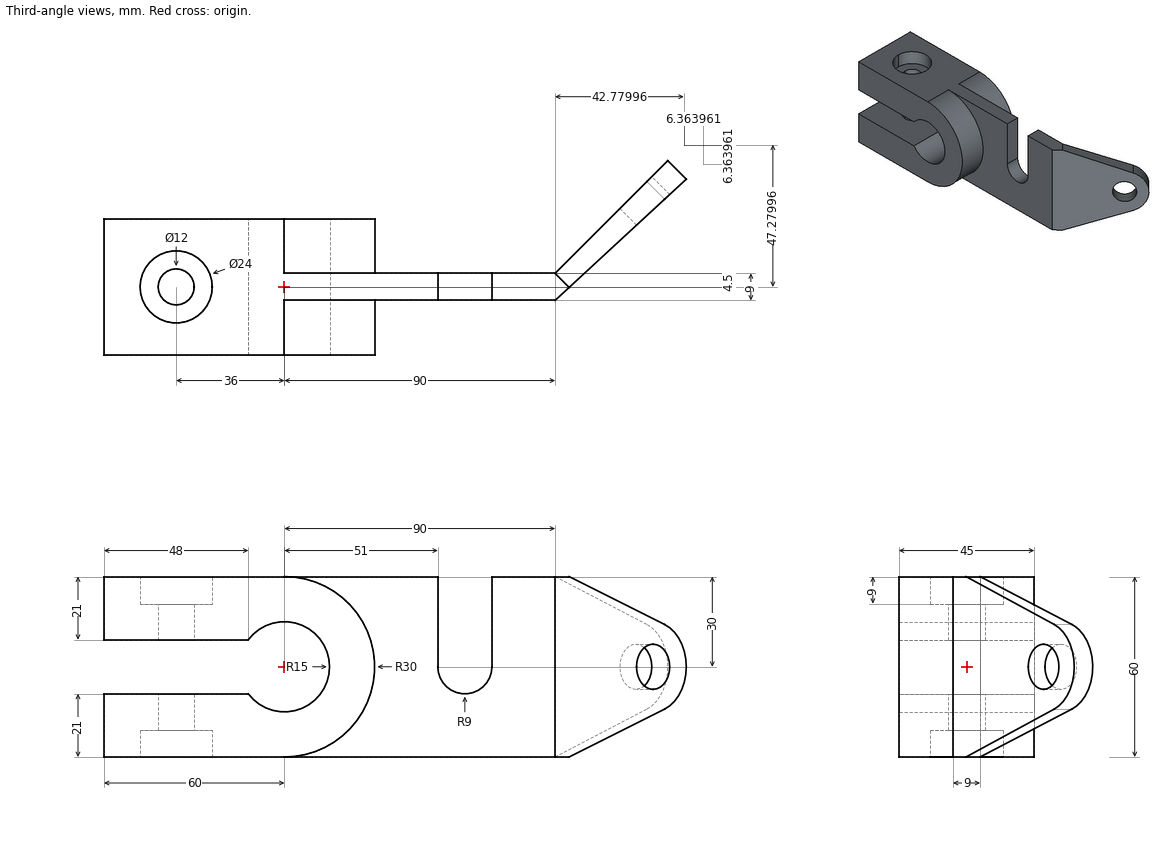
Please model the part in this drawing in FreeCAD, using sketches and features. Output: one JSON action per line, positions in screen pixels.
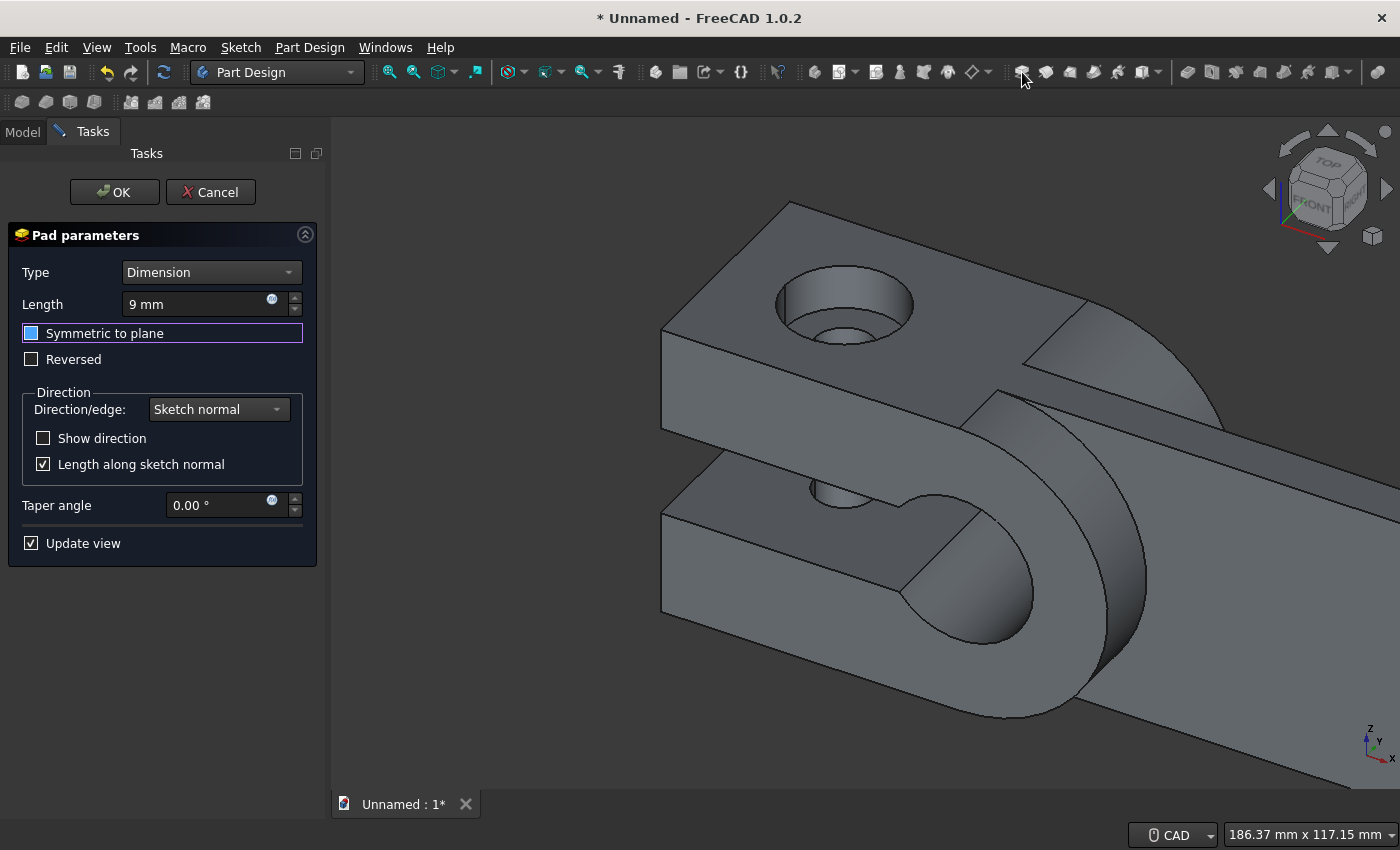
{"action": "left_click", "coordinate": [30, 333]}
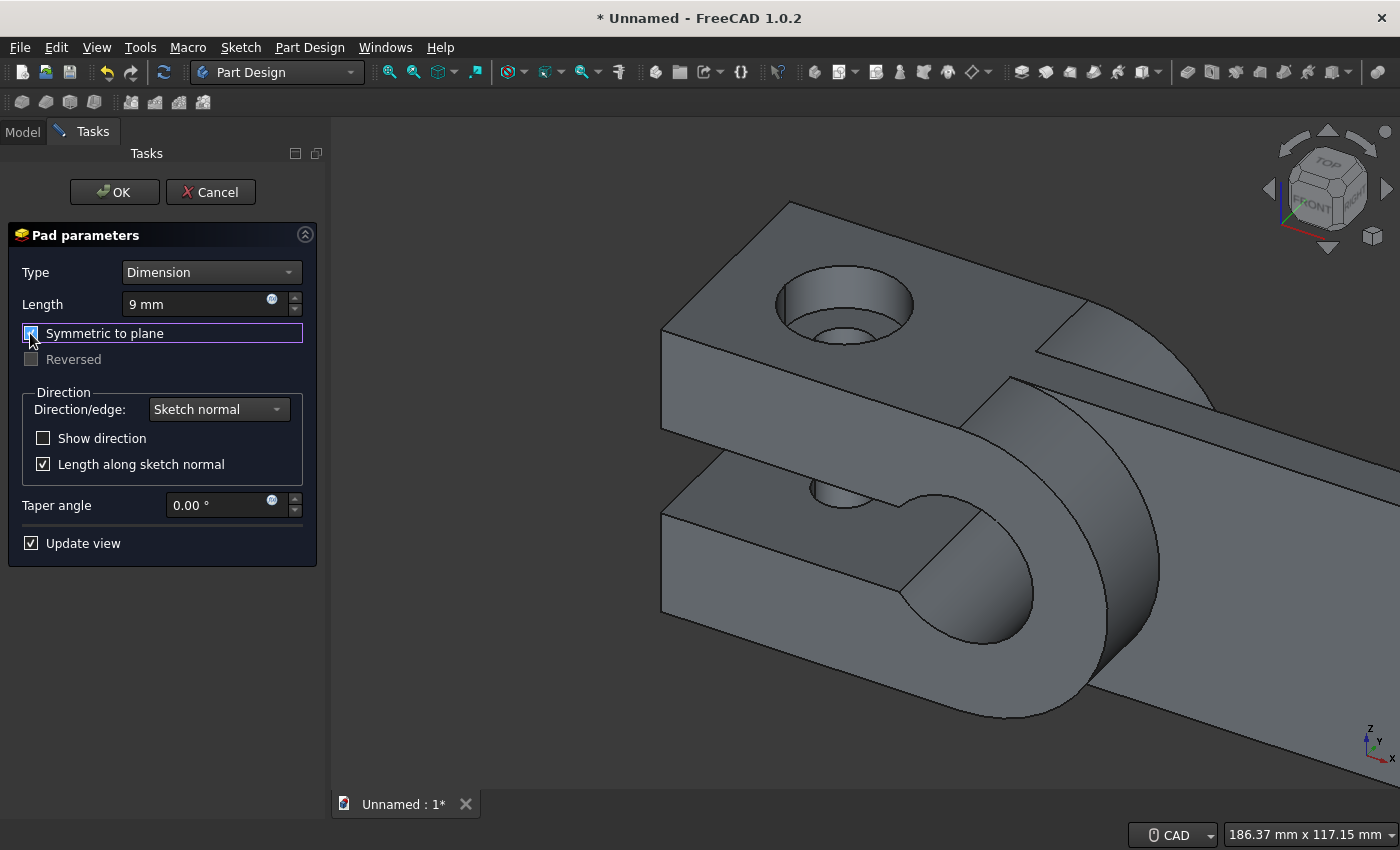
{"action": "left_click", "coordinate": [115, 192]}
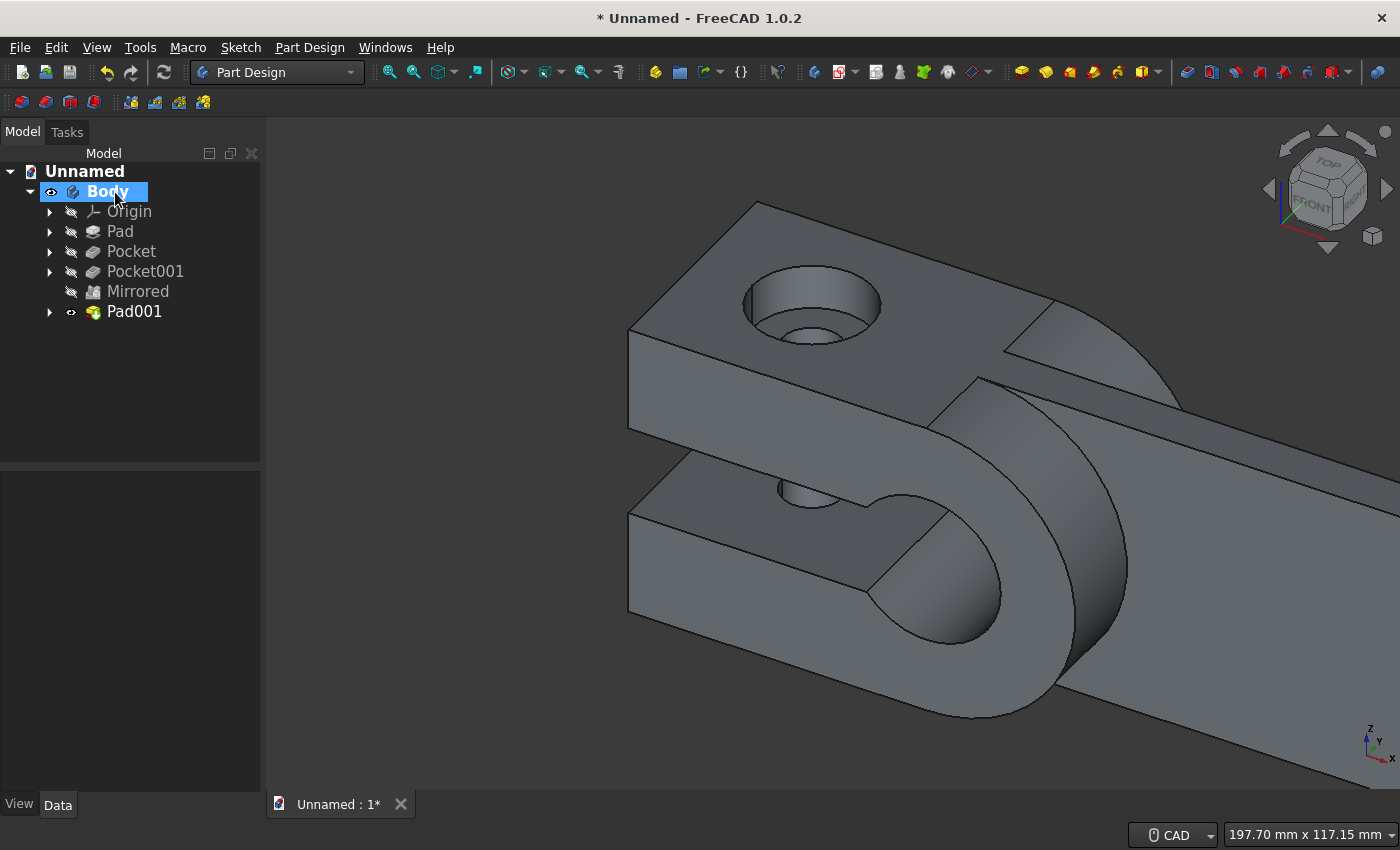
{"action": "key", "text": "v f"}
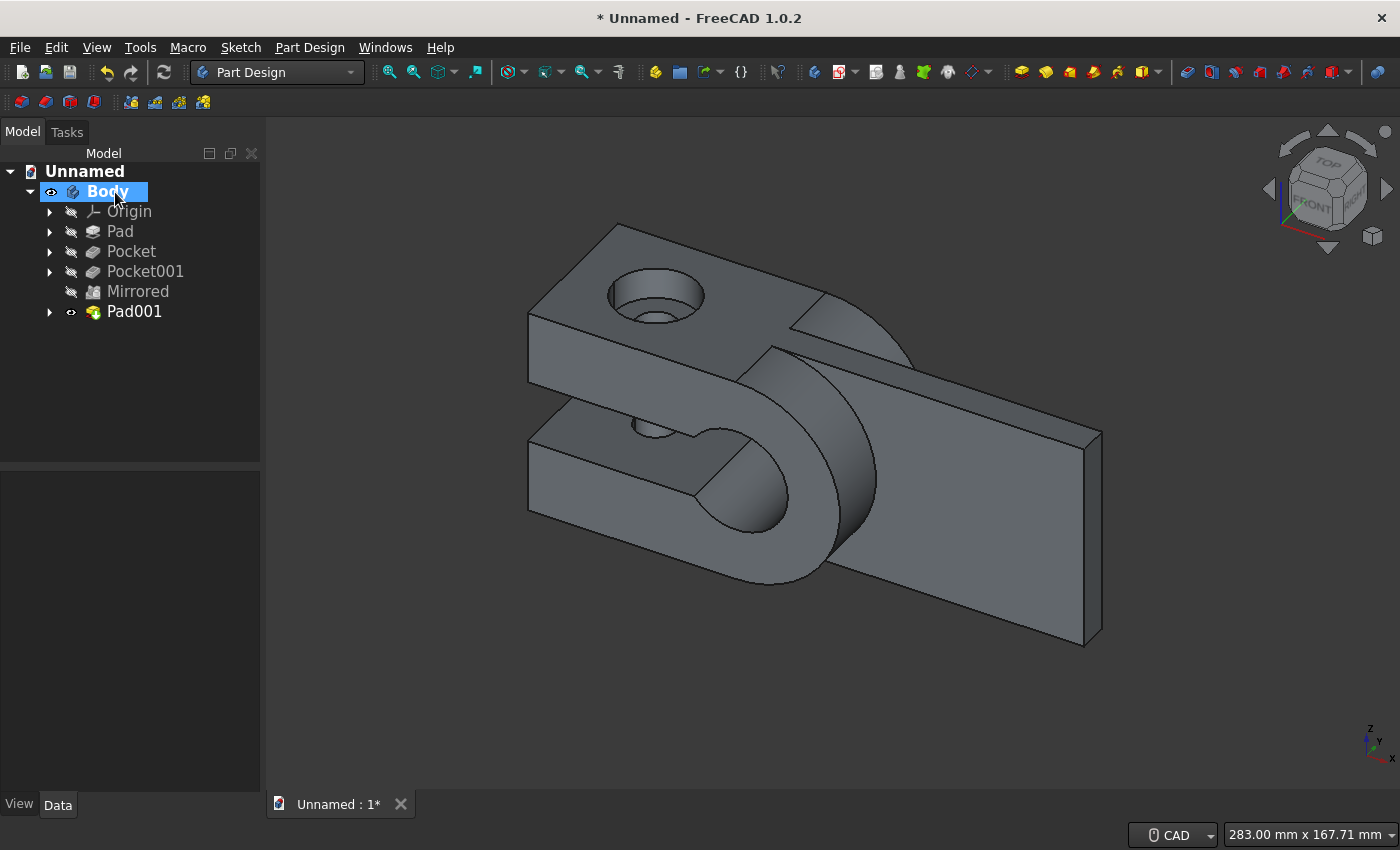
{"action": "left_click", "coordinate": [759, 329]}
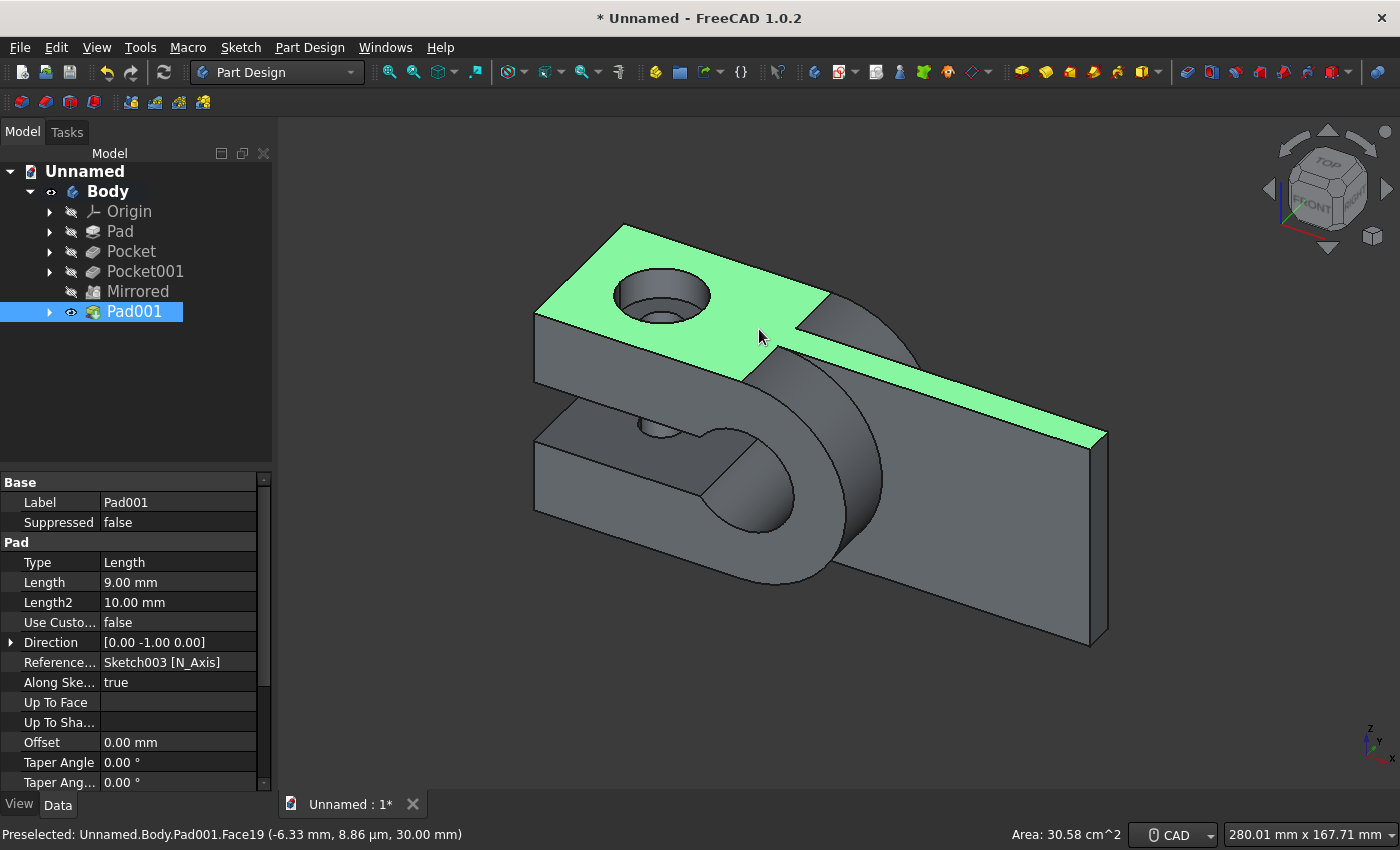
{"action": "left_click", "coordinate": [840, 72]}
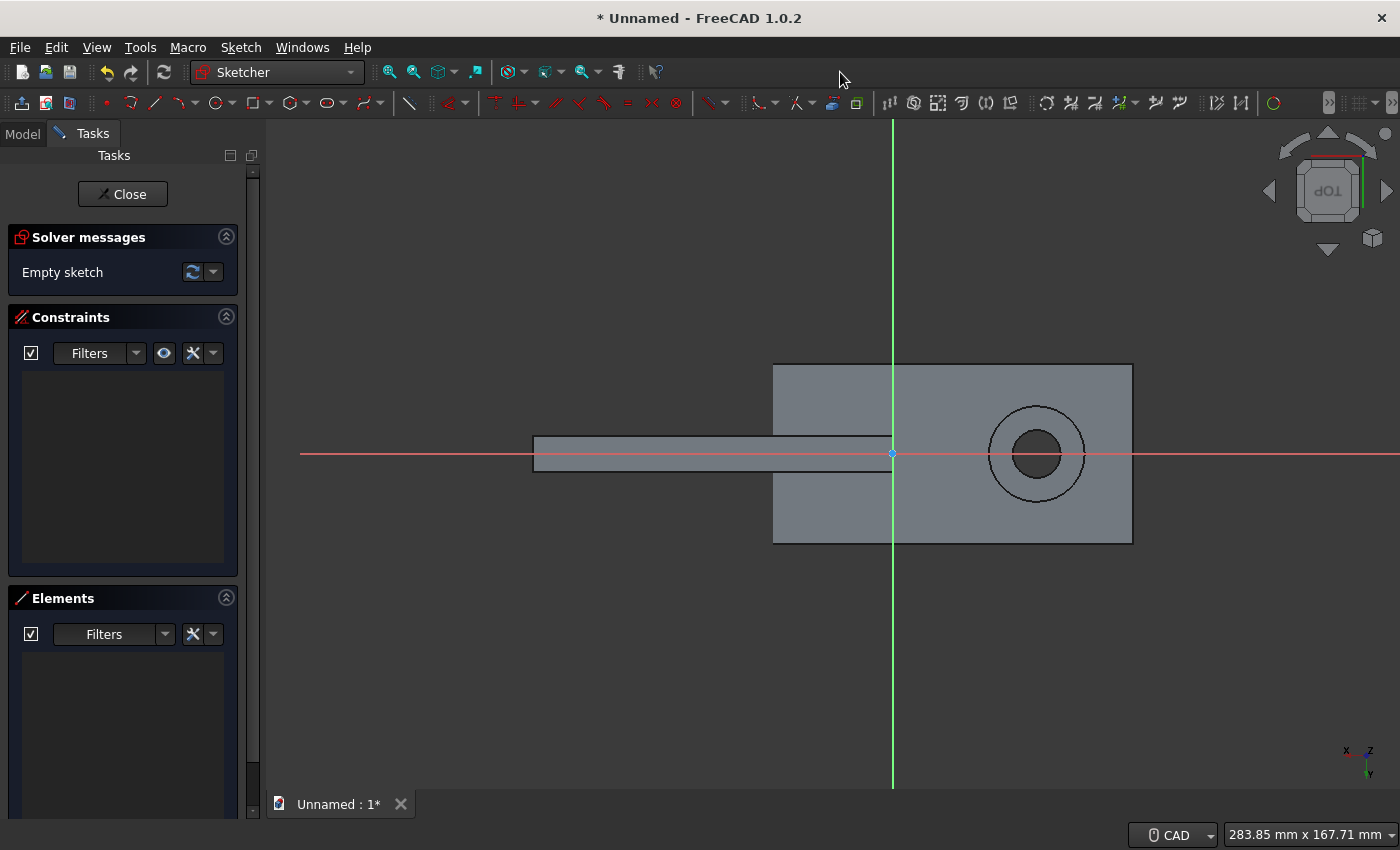
{"action": "scroll", "coordinate": [294, 609], "scroll_direction": "up", "scroll_amount": 4}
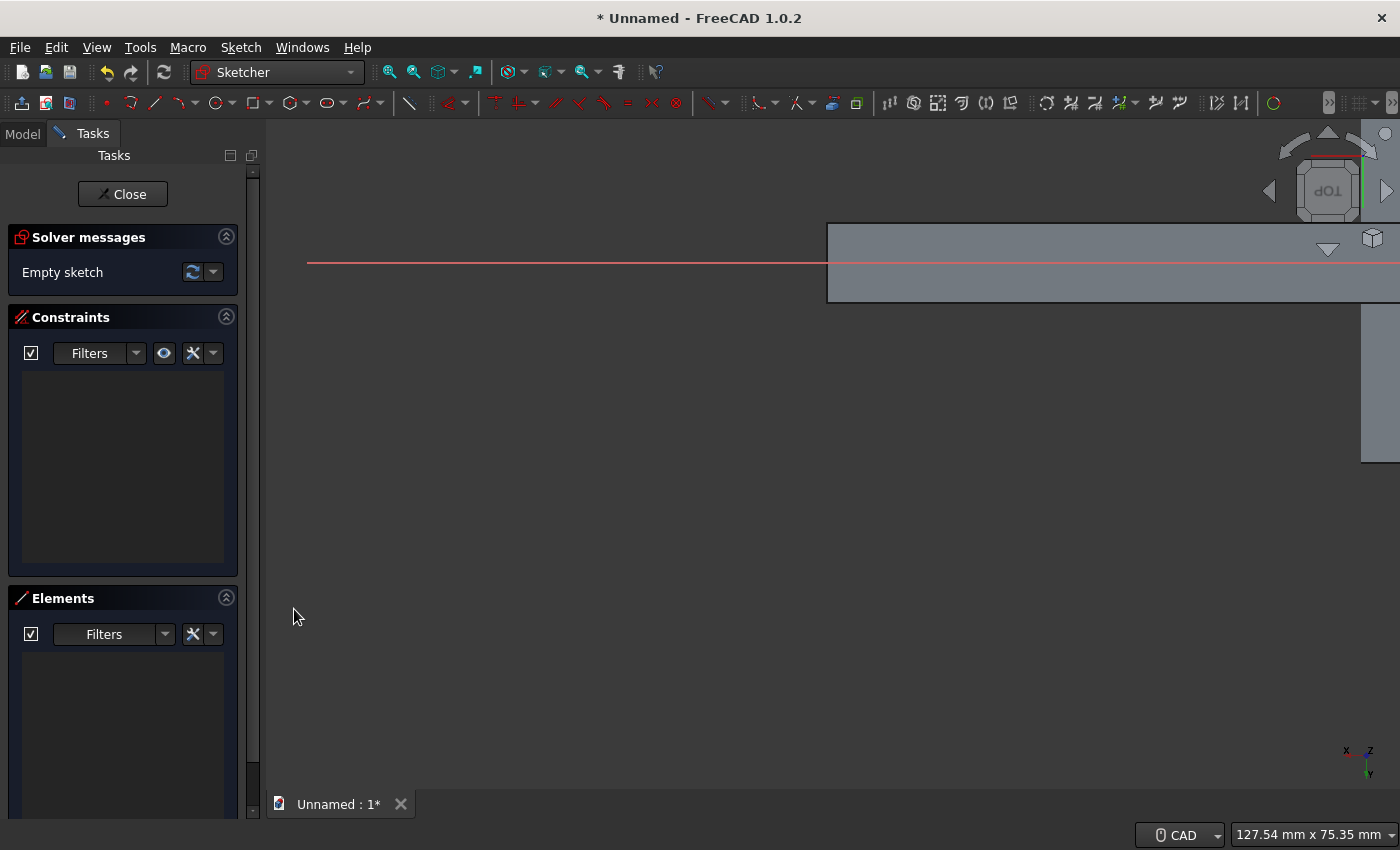
{"action": "left_click", "coordinate": [132, 104]}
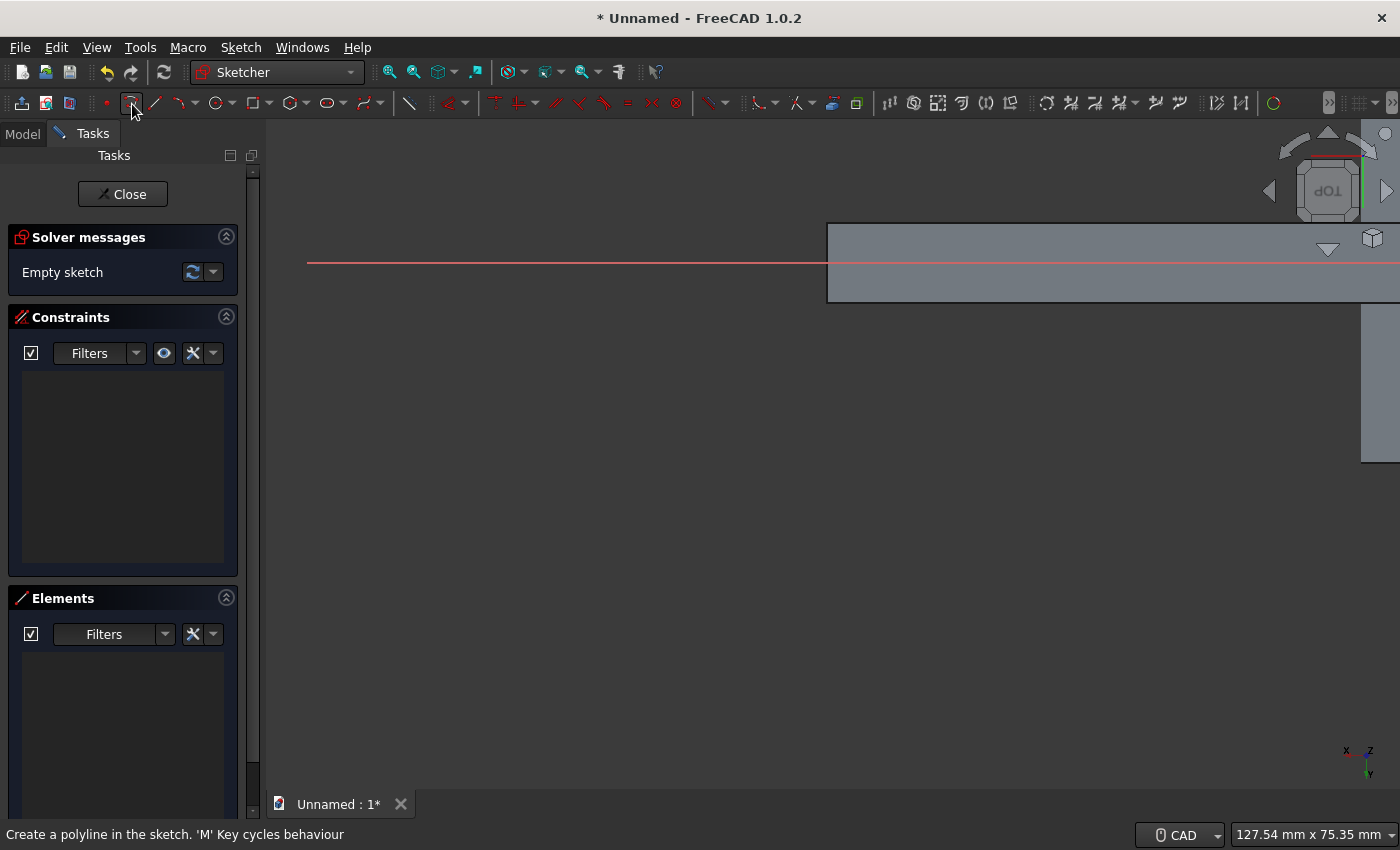
{"action": "left_click", "coordinate": [827, 303]}
{"action": "left_click", "coordinate": [827, 223]}
{"action": "left_click", "coordinate": [390, 627]}
{"action": "left_click", "coordinate": [446, 684]}
{"action": "left_click", "coordinate": [827, 304]}
{"action": "key", "text": "Escape"}
{"action": "key", "text": "Escape"}